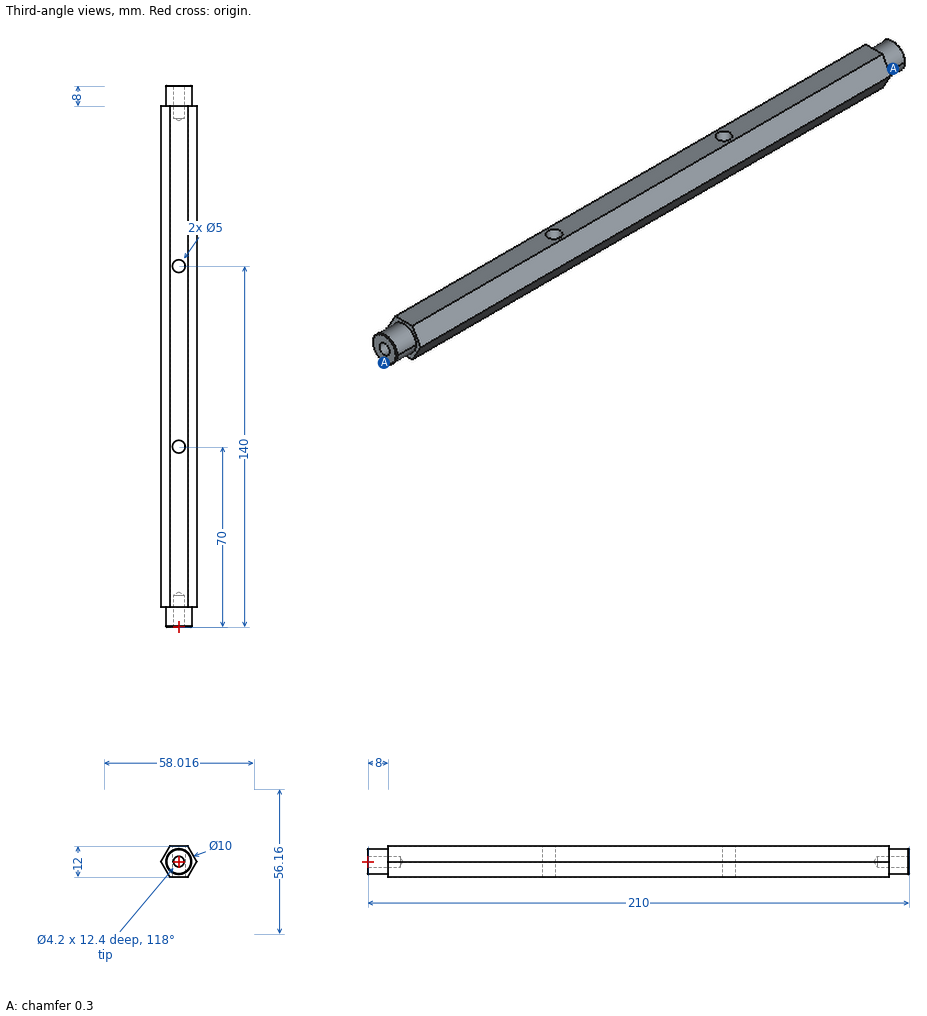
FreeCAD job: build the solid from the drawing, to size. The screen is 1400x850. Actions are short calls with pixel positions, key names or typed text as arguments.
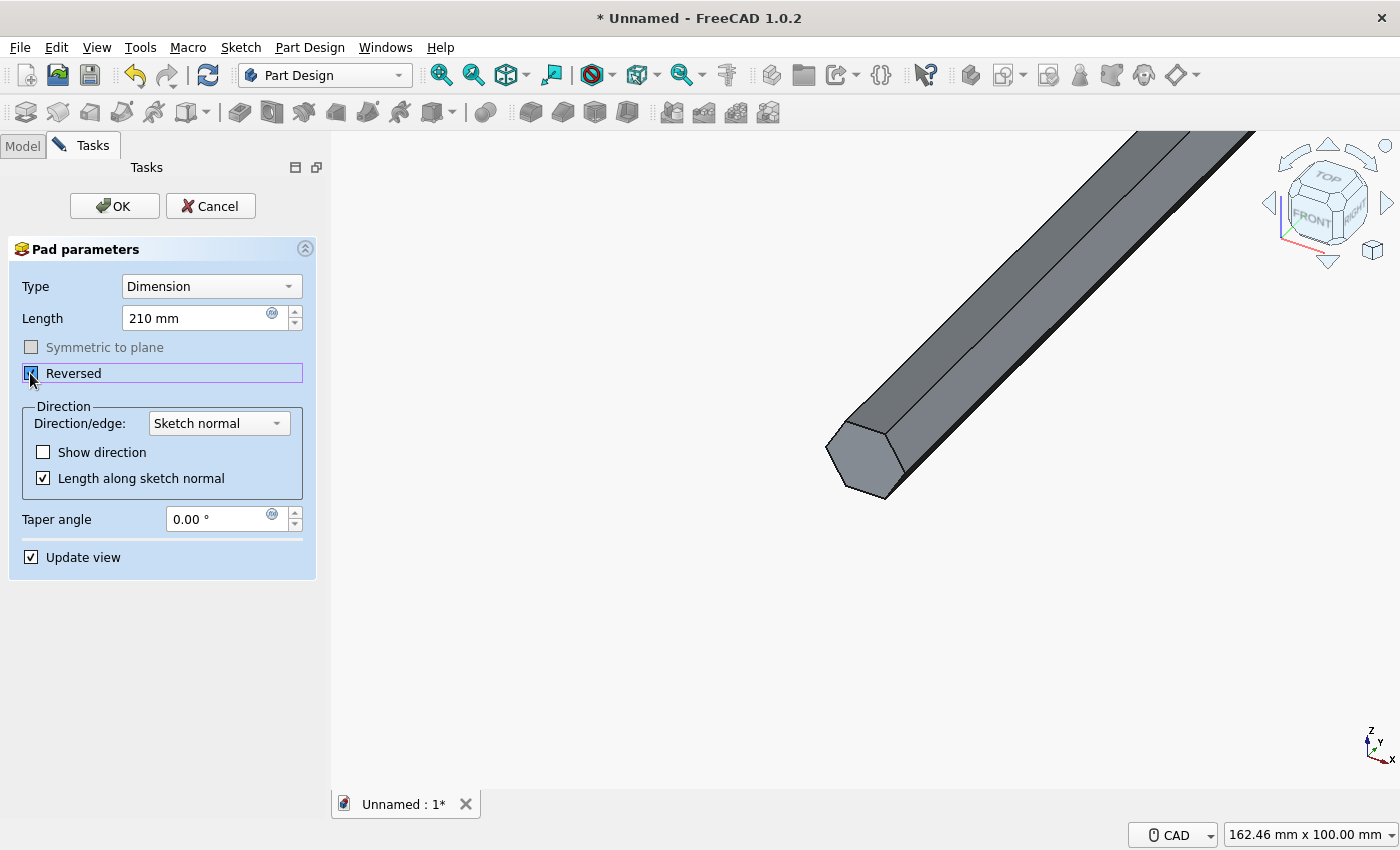
click(115, 206)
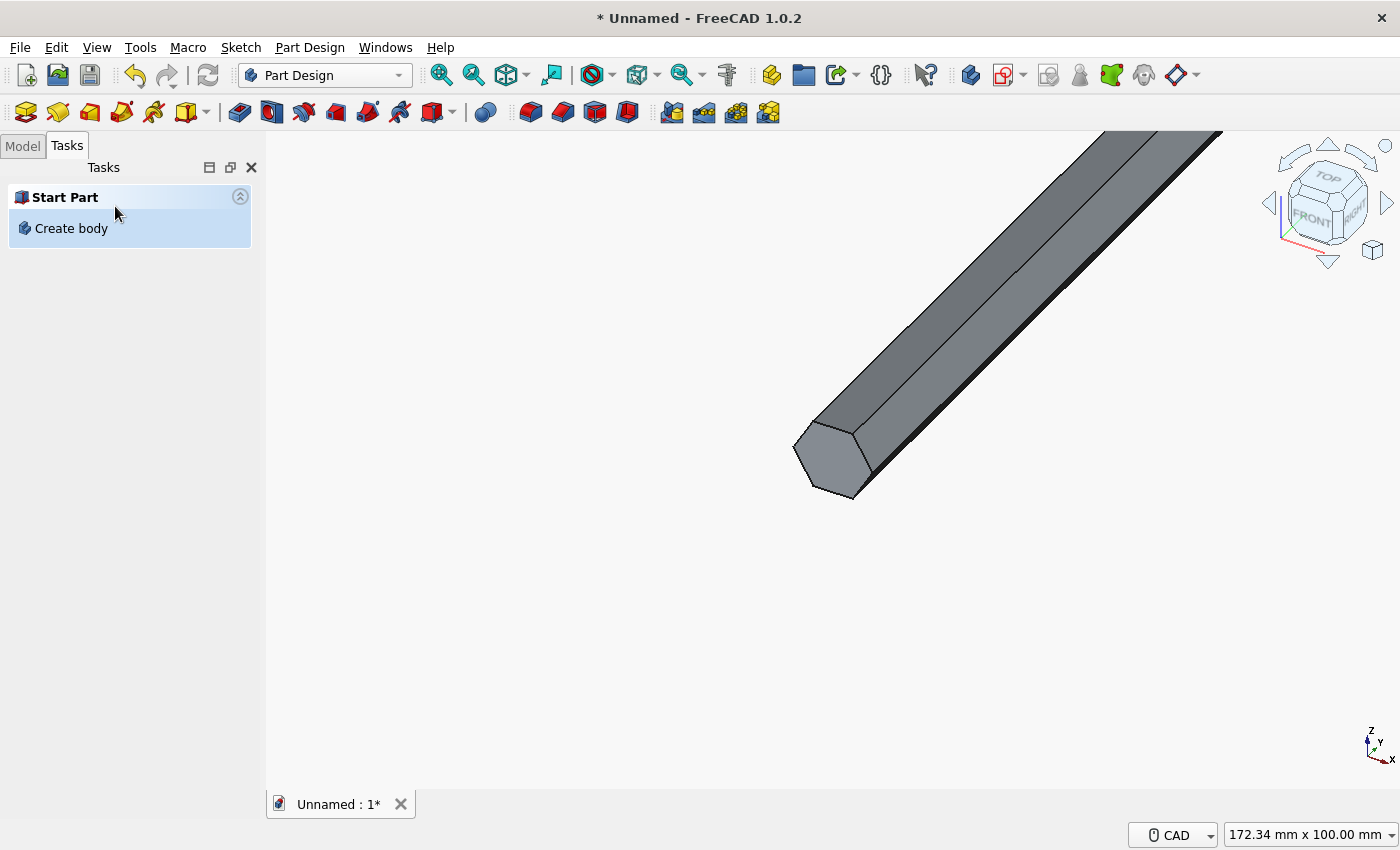
key(v)
key(f)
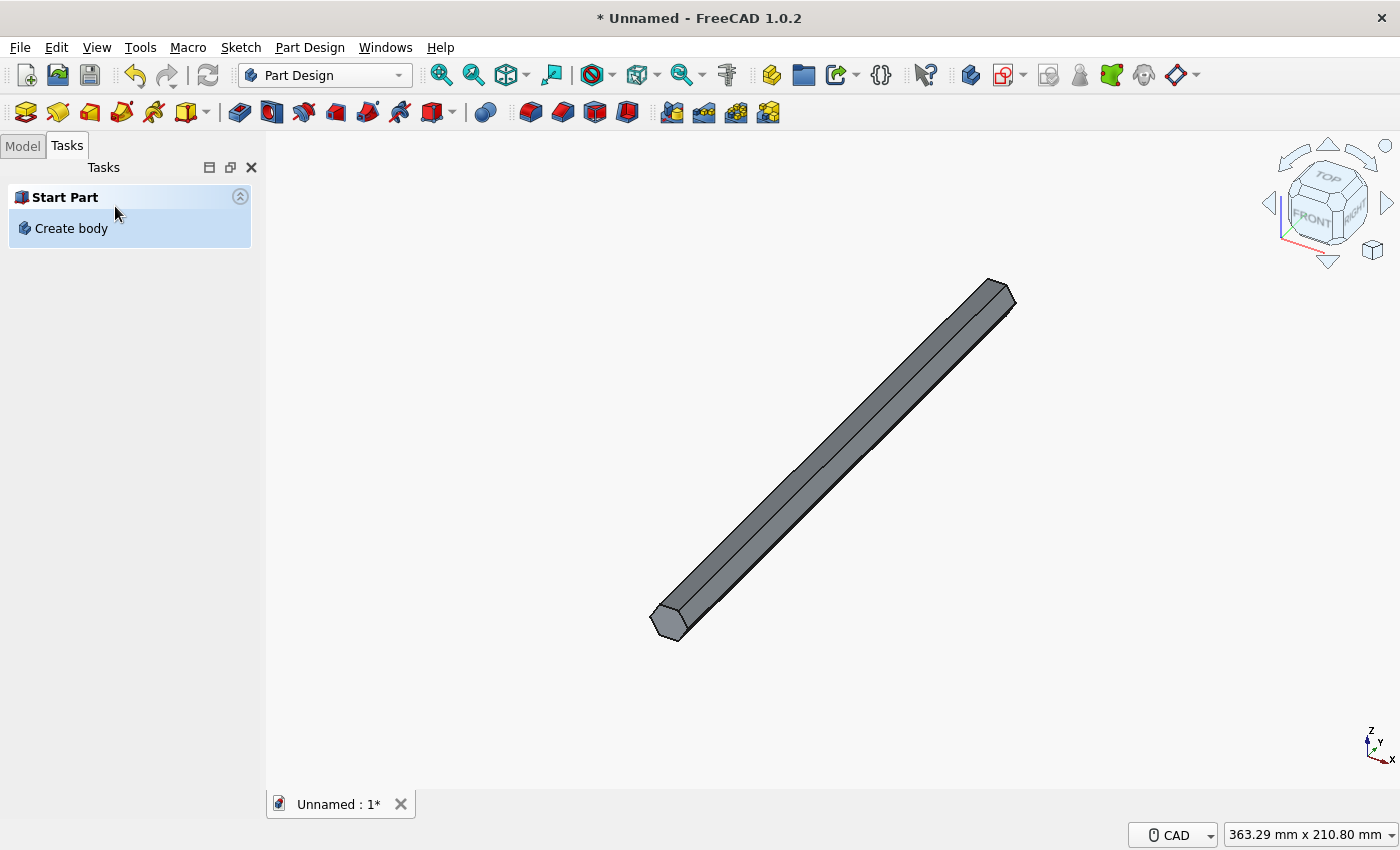
key(4)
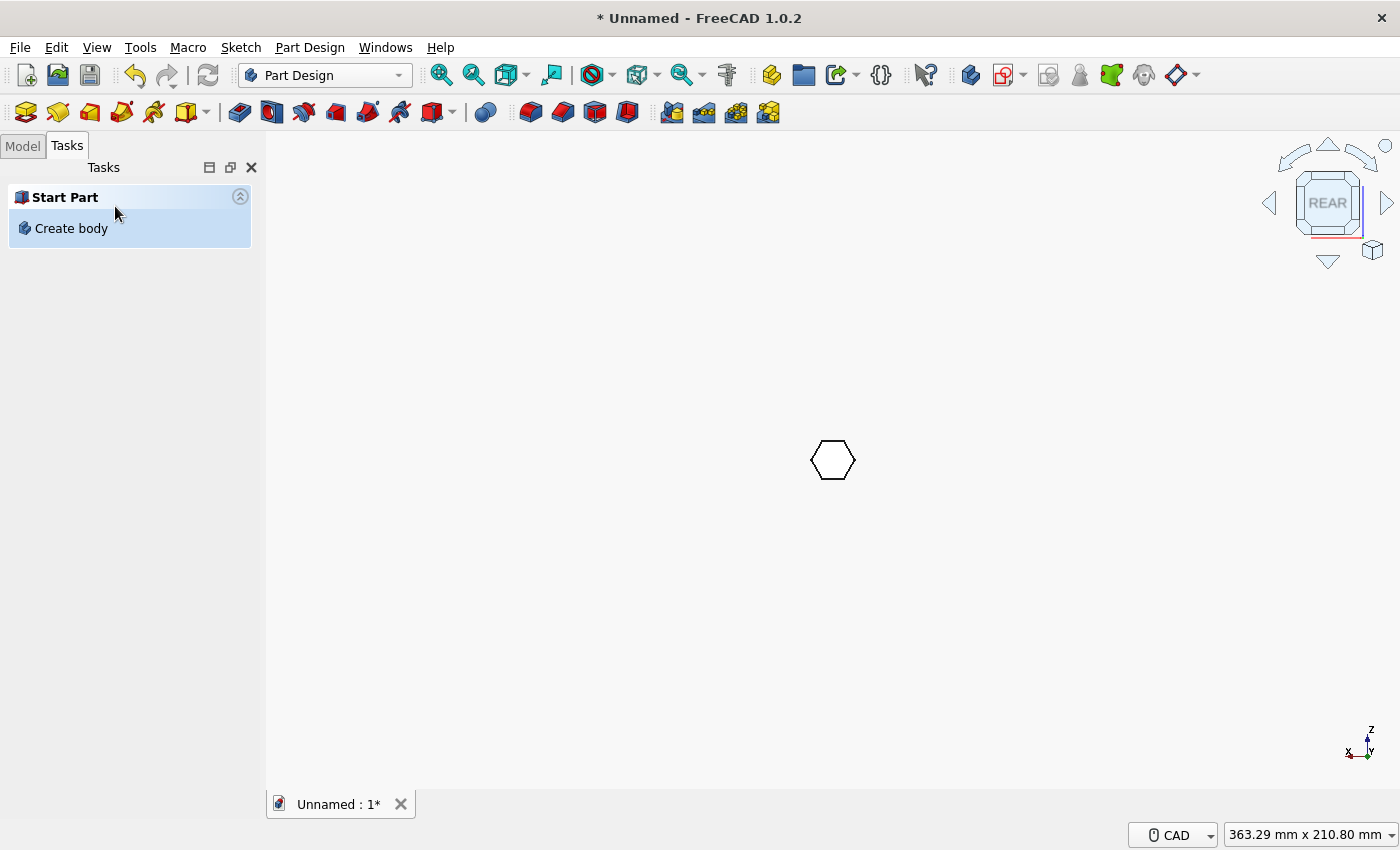
click(442, 76)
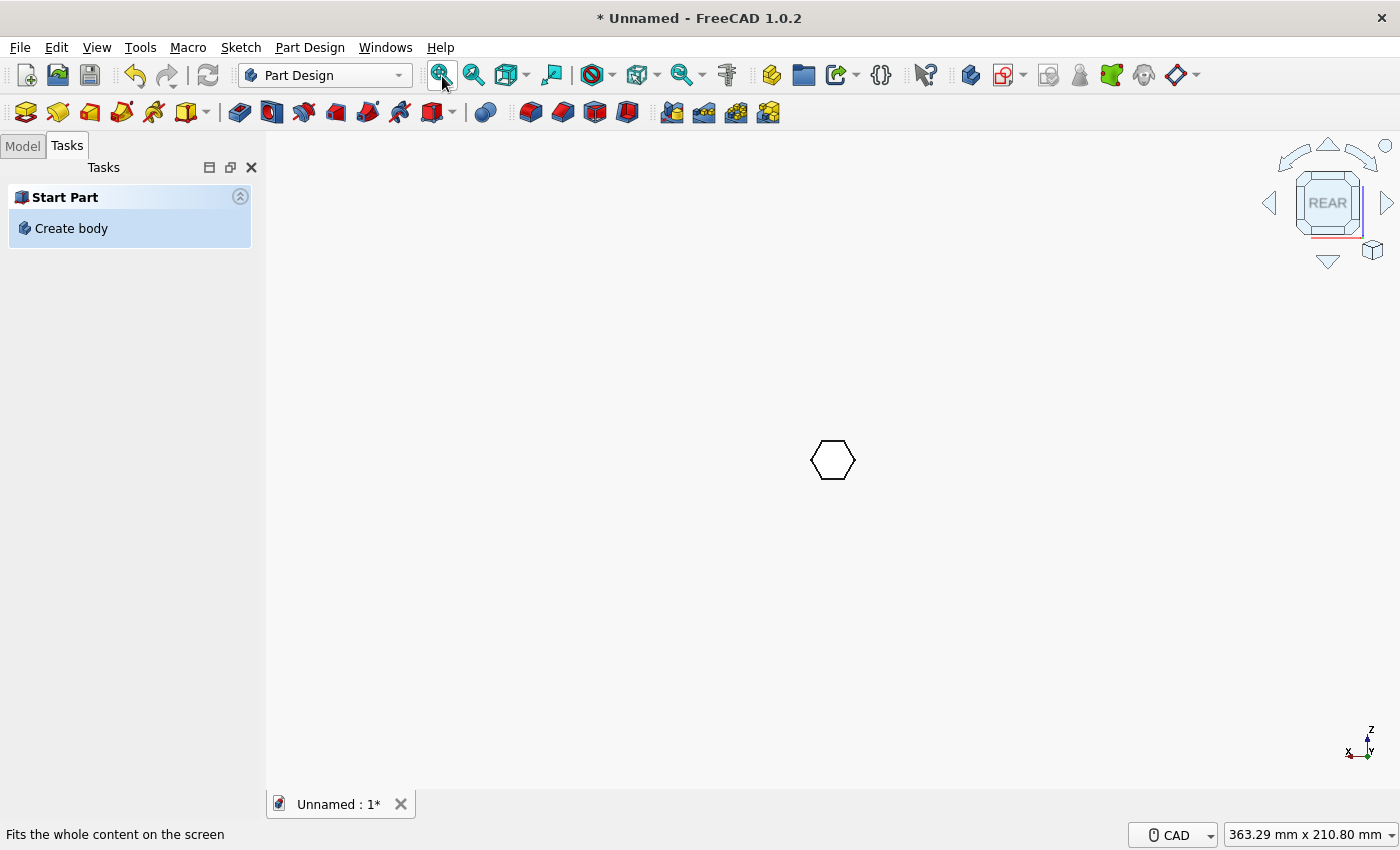
click(833, 459)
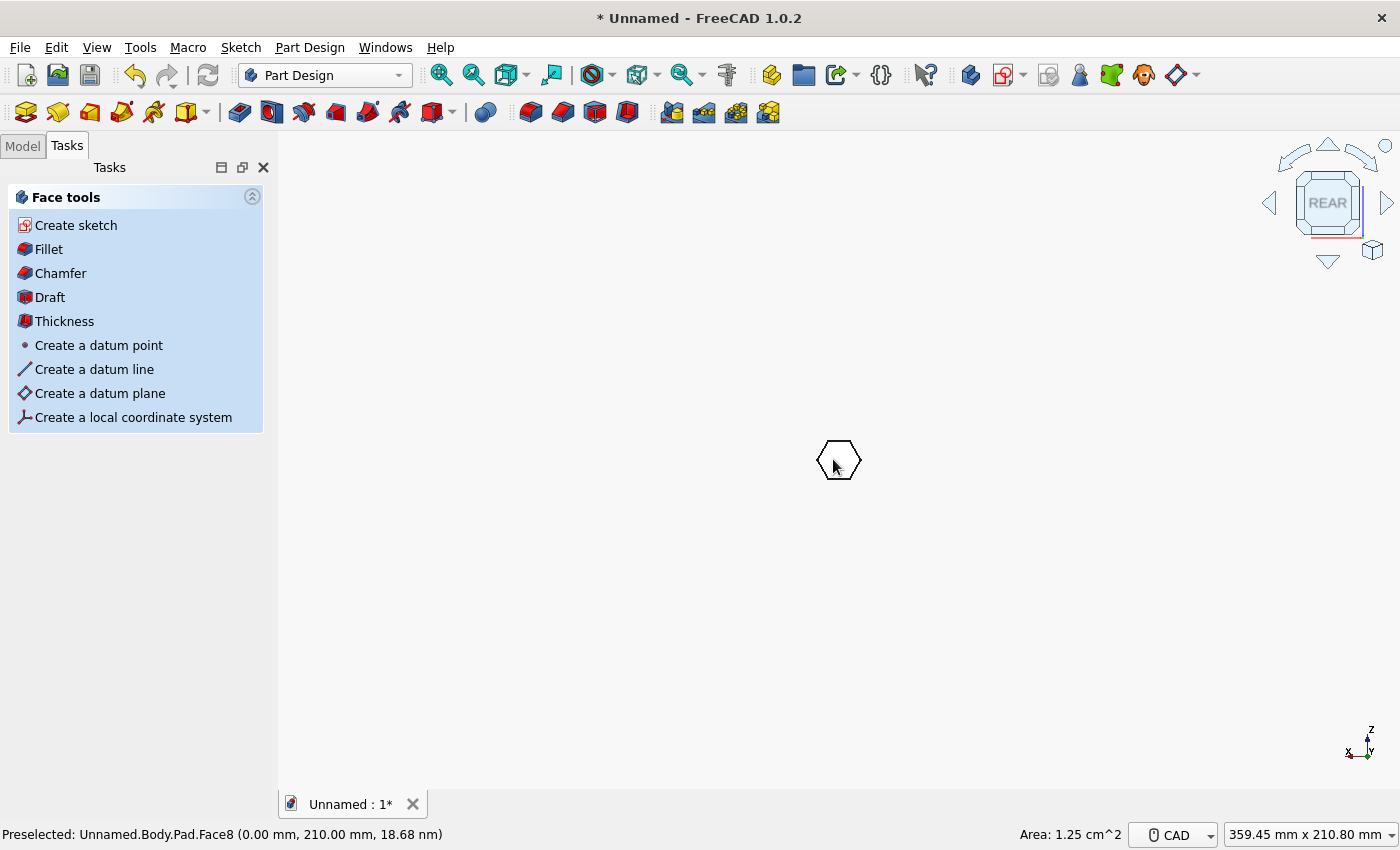
click(1004, 76)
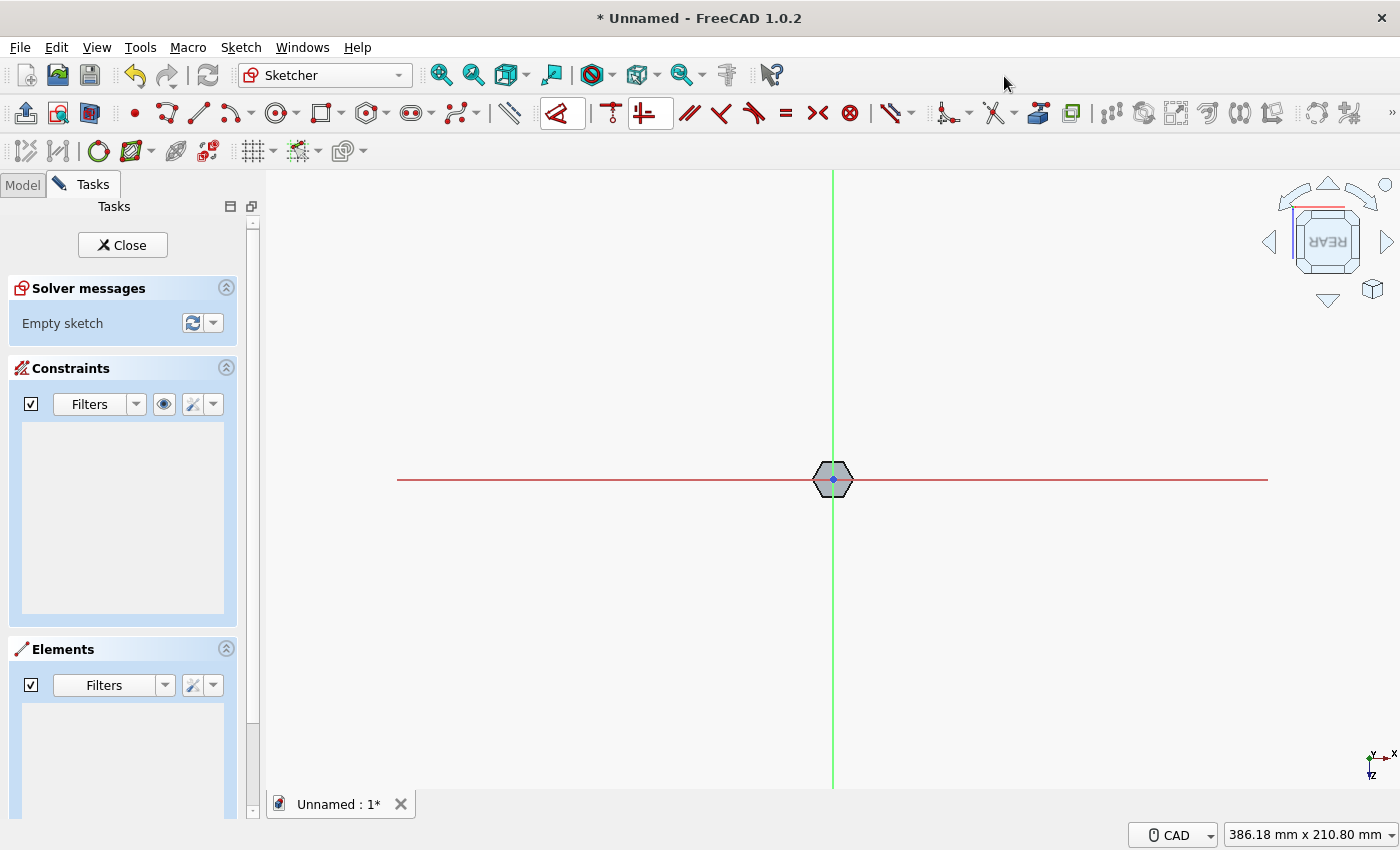
scroll(889, 479, up, 4)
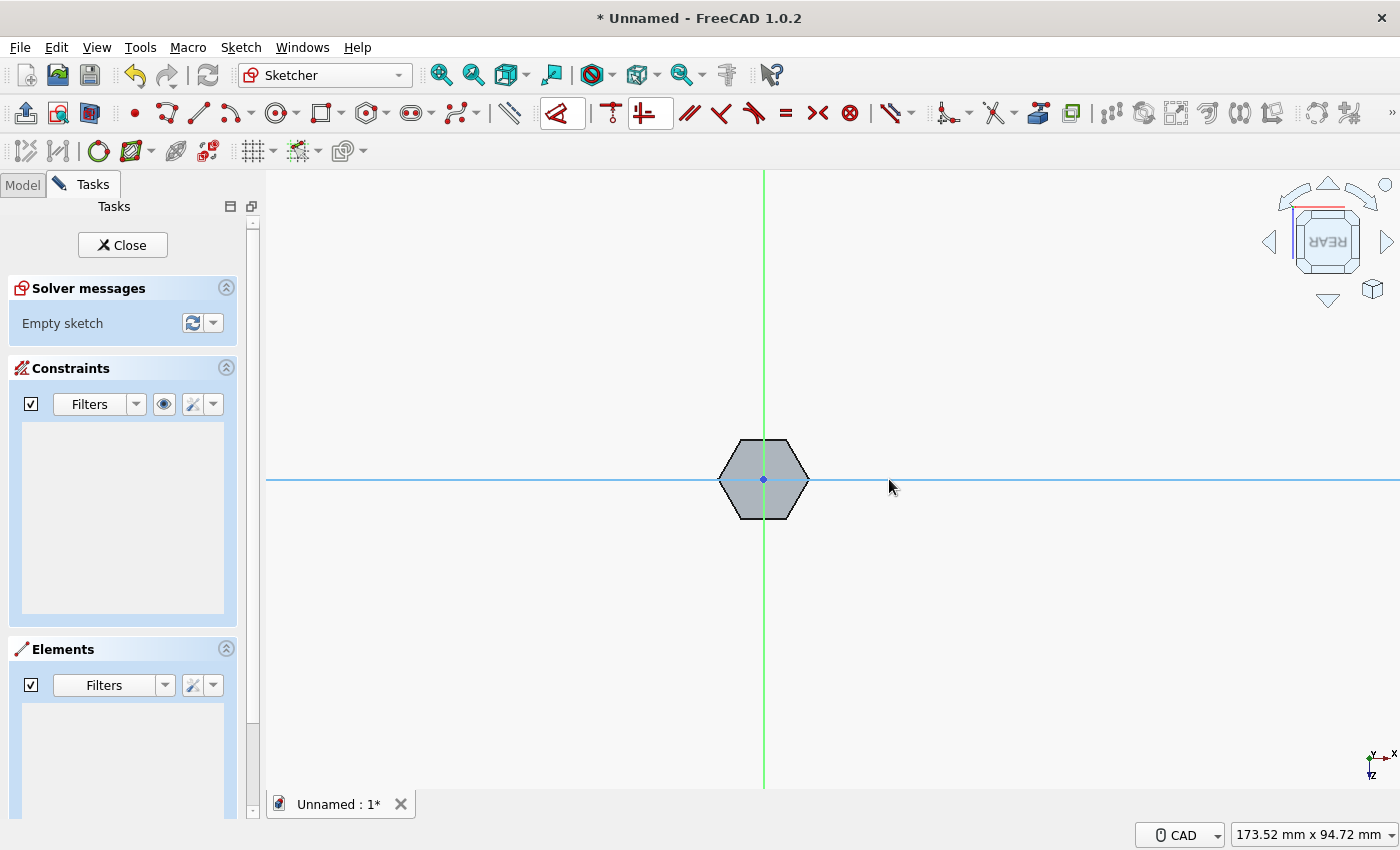
key(g)
key(v)